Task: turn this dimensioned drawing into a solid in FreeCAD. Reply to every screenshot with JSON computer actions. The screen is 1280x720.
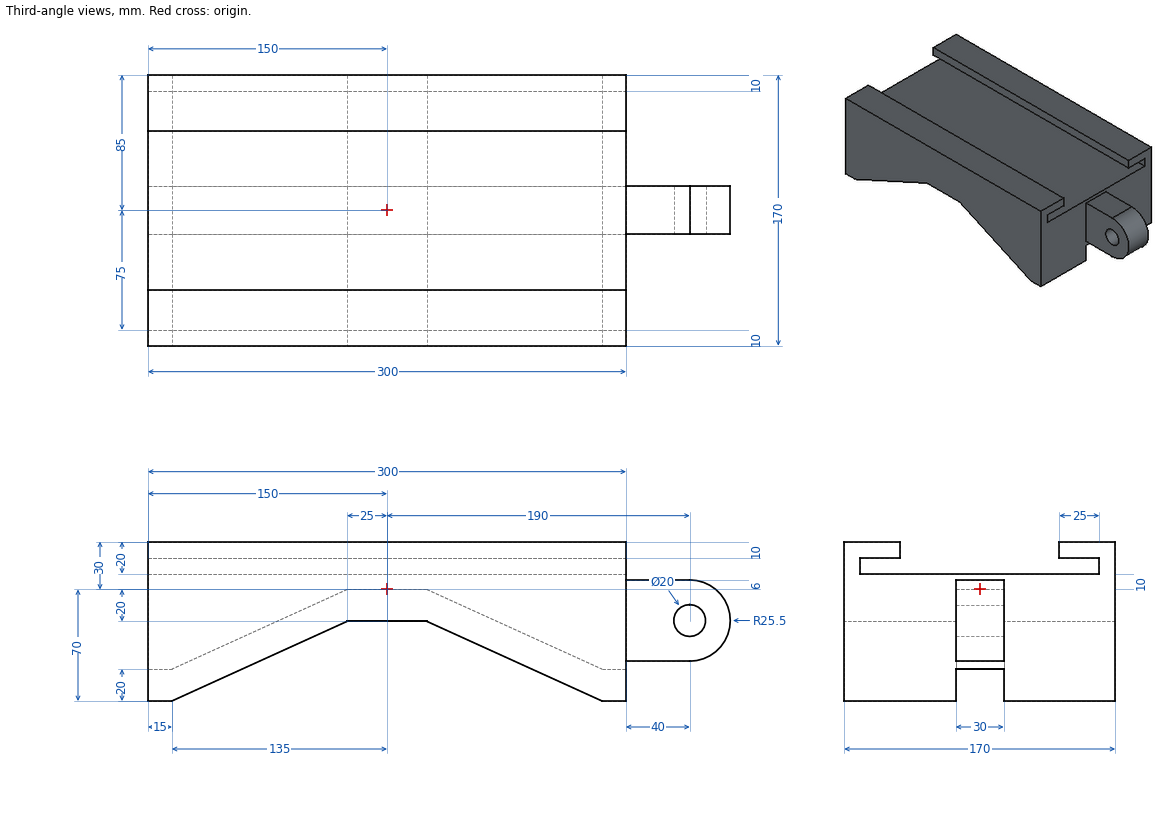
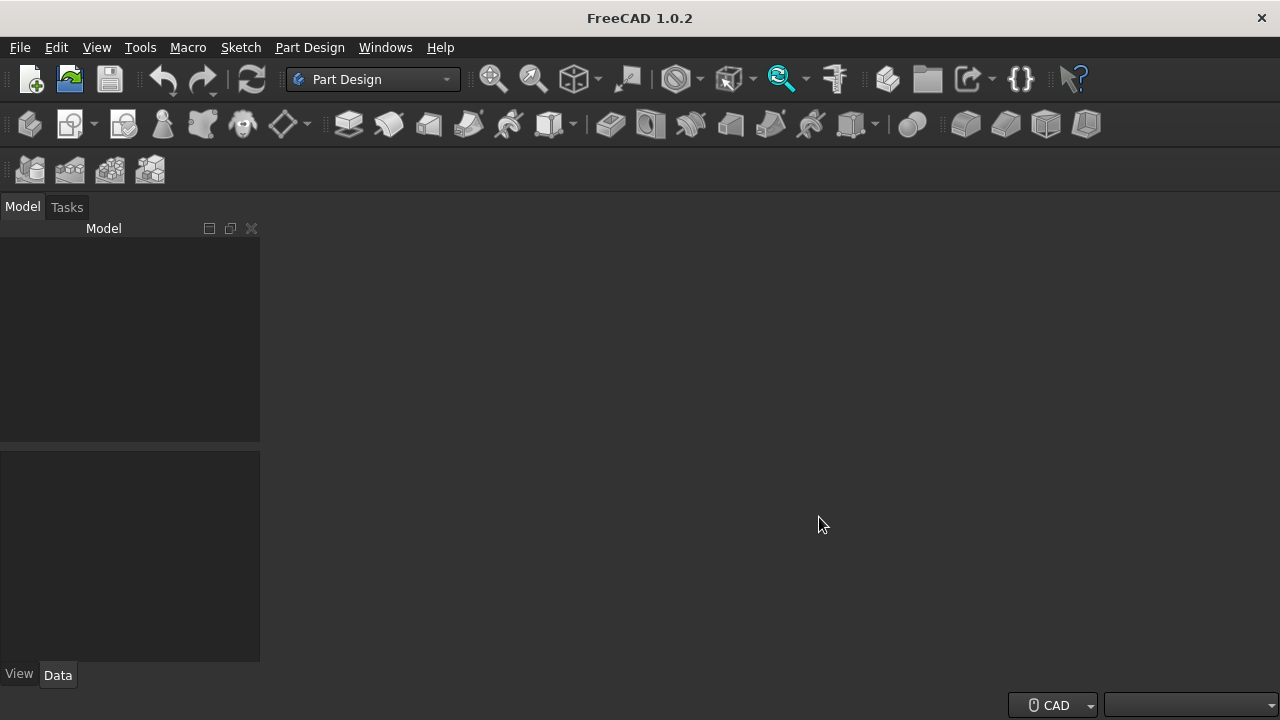
{"action": "left_click", "coordinate": [30, 80]}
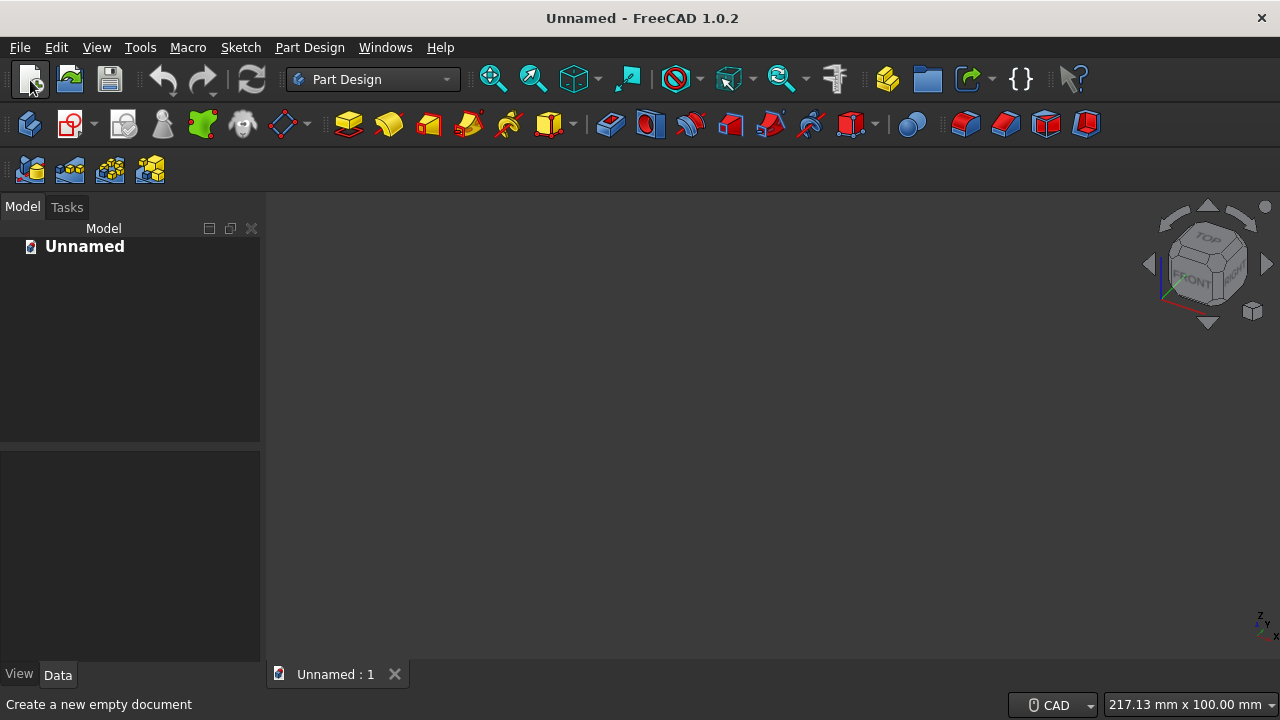
{"action": "left_click", "coordinate": [70, 124]}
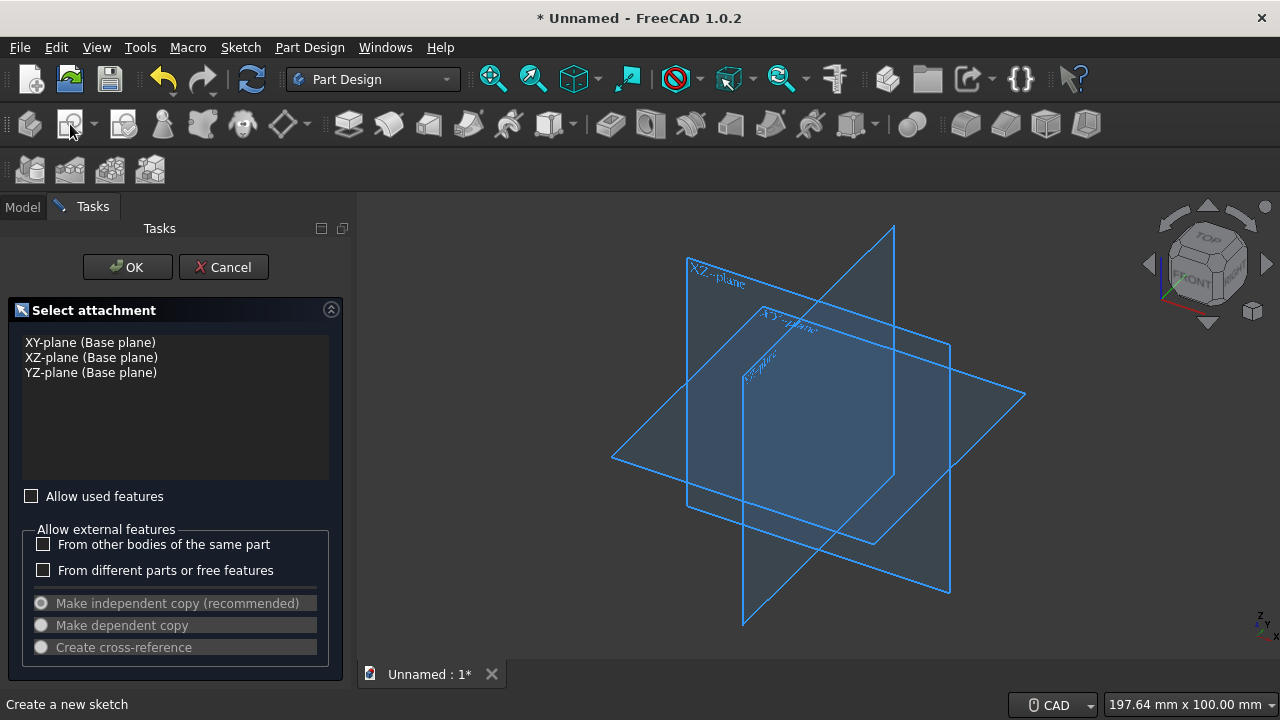
{"action": "left_click", "coordinate": [82, 342]}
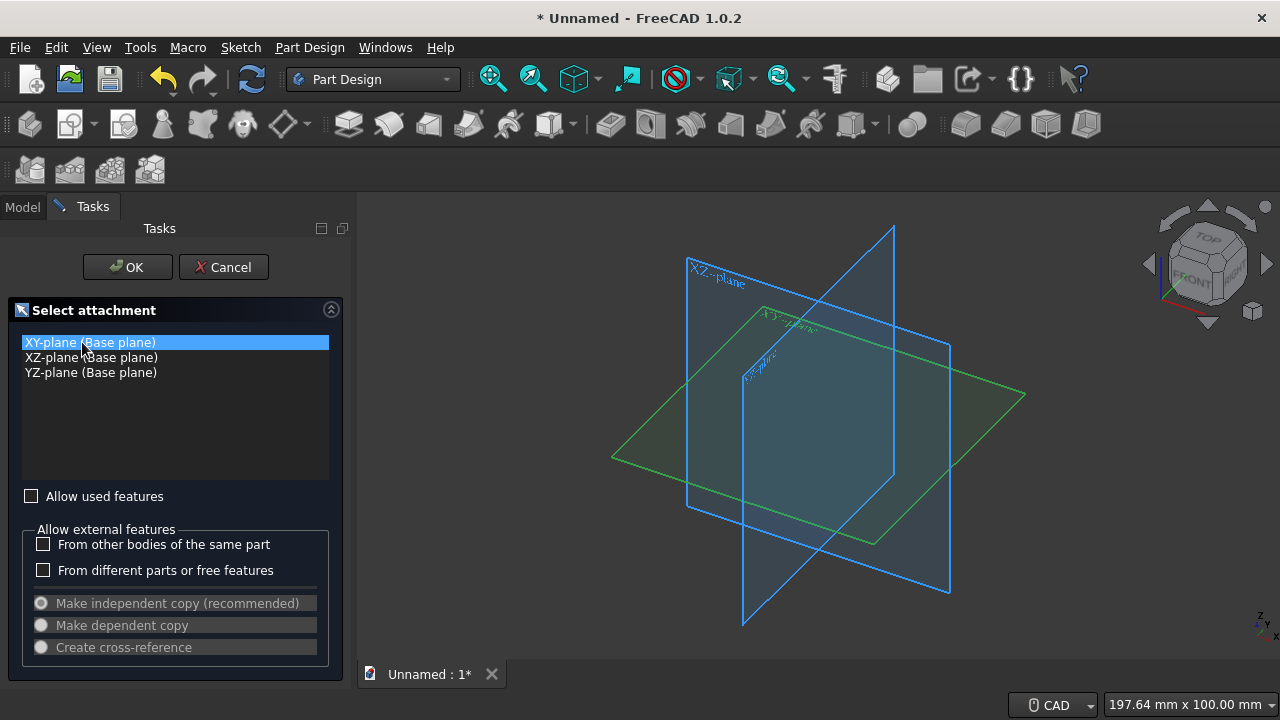
{"action": "left_click", "coordinate": [128, 267]}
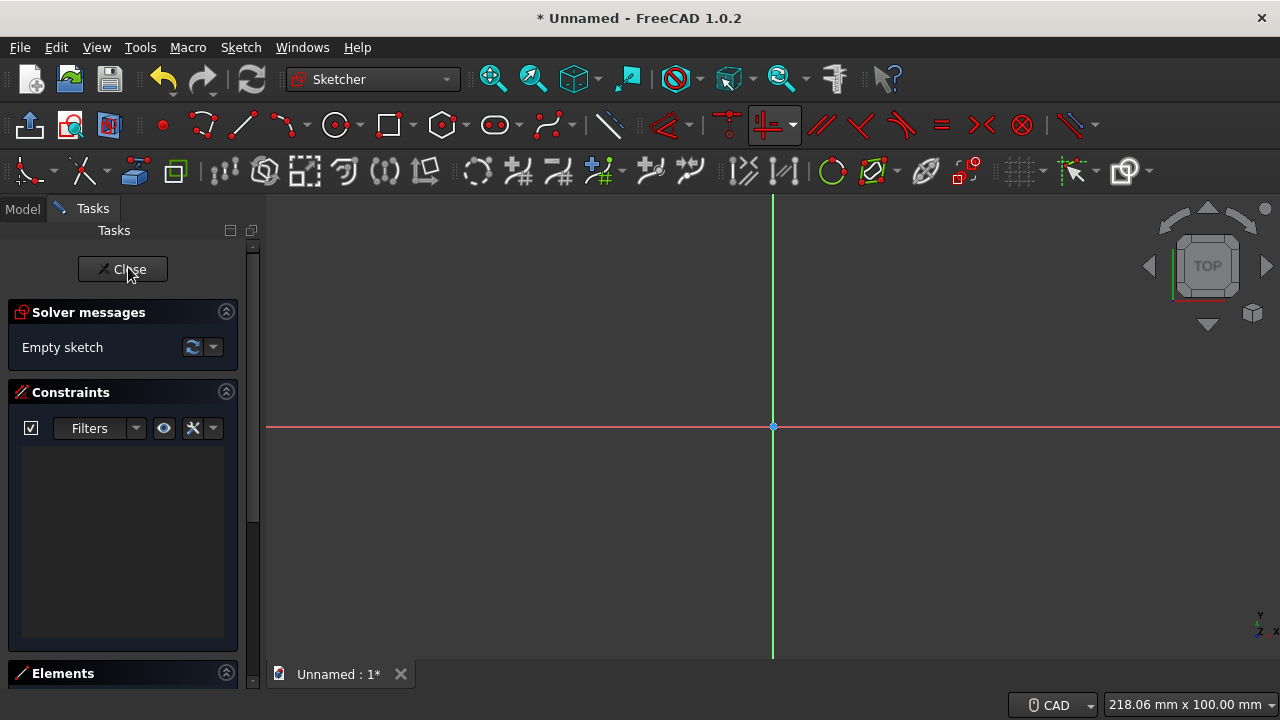
{"action": "scroll", "coordinate": [665, 427], "scroll_direction": "down", "scroll_amount": 5}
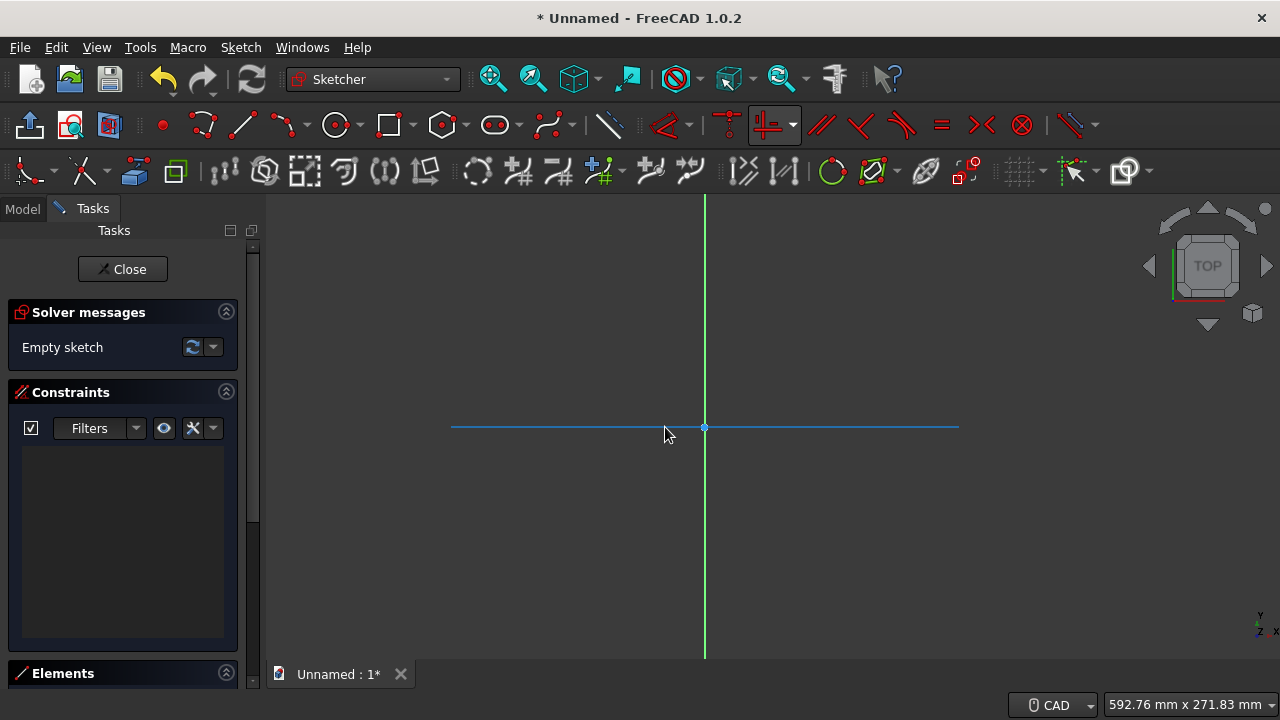
{"action": "key", "text": "g v"}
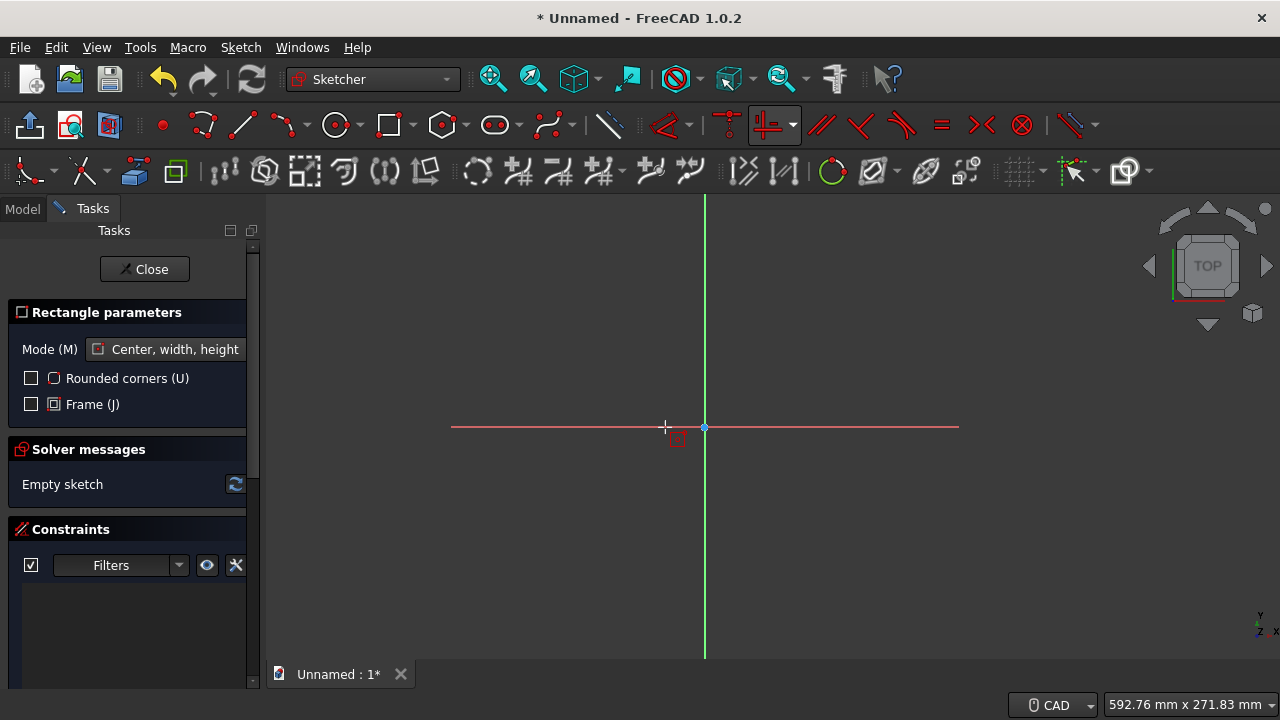
{"action": "left_click", "coordinate": [705, 427]}
{"action": "mouse_move", "coordinate": [962, 282]}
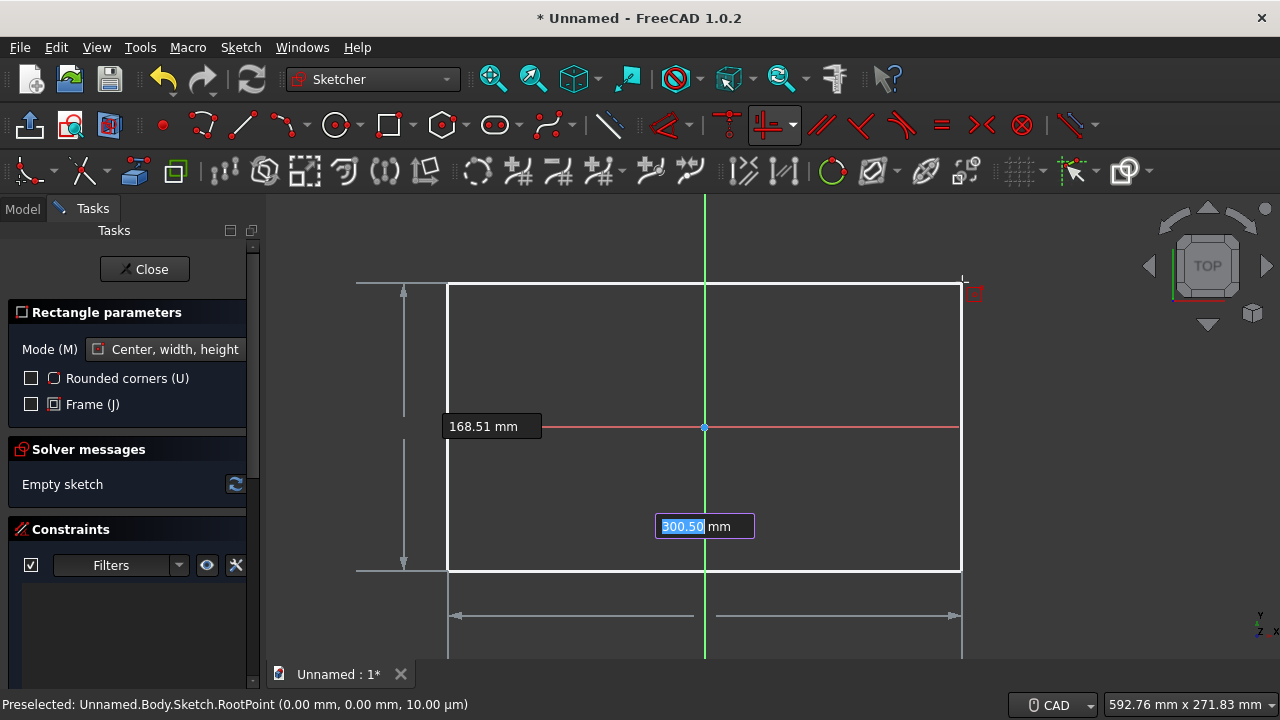
{"action": "type", "text": "300"}
{"action": "key", "text": "Tab"}
{"action": "type", "text": "170"}
{"action": "key", "text": "Return"}
{"action": "key", "text": "Escape"}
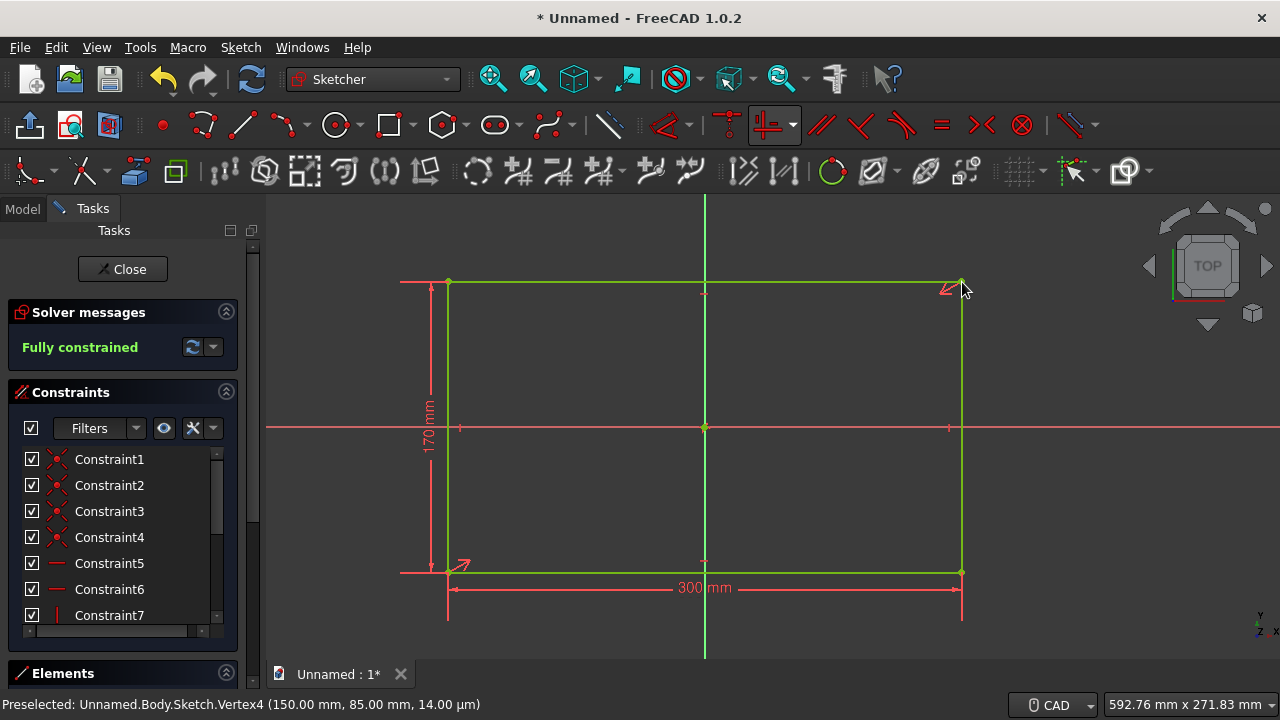
{"action": "left_click", "coordinate": [123, 269]}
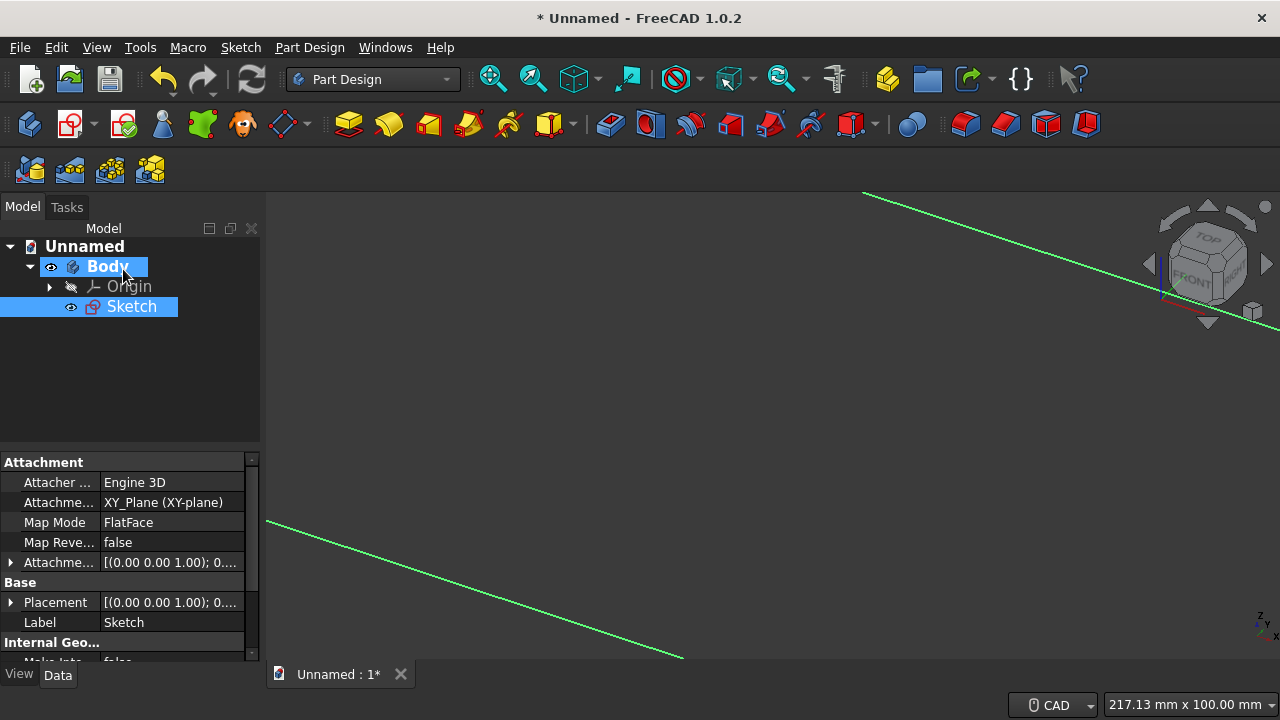
{"action": "left_click", "coordinate": [350, 124]}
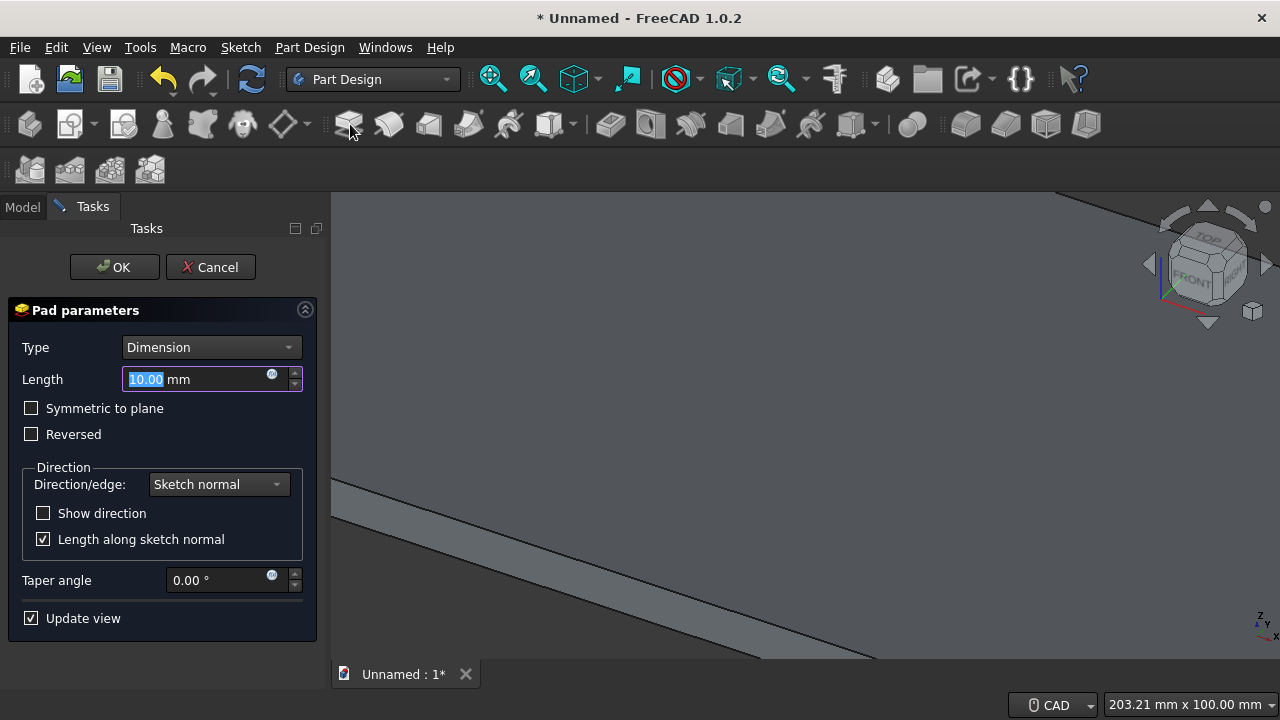
{"action": "type", "text": "10"}
{"action": "key", "text": "Tab"}